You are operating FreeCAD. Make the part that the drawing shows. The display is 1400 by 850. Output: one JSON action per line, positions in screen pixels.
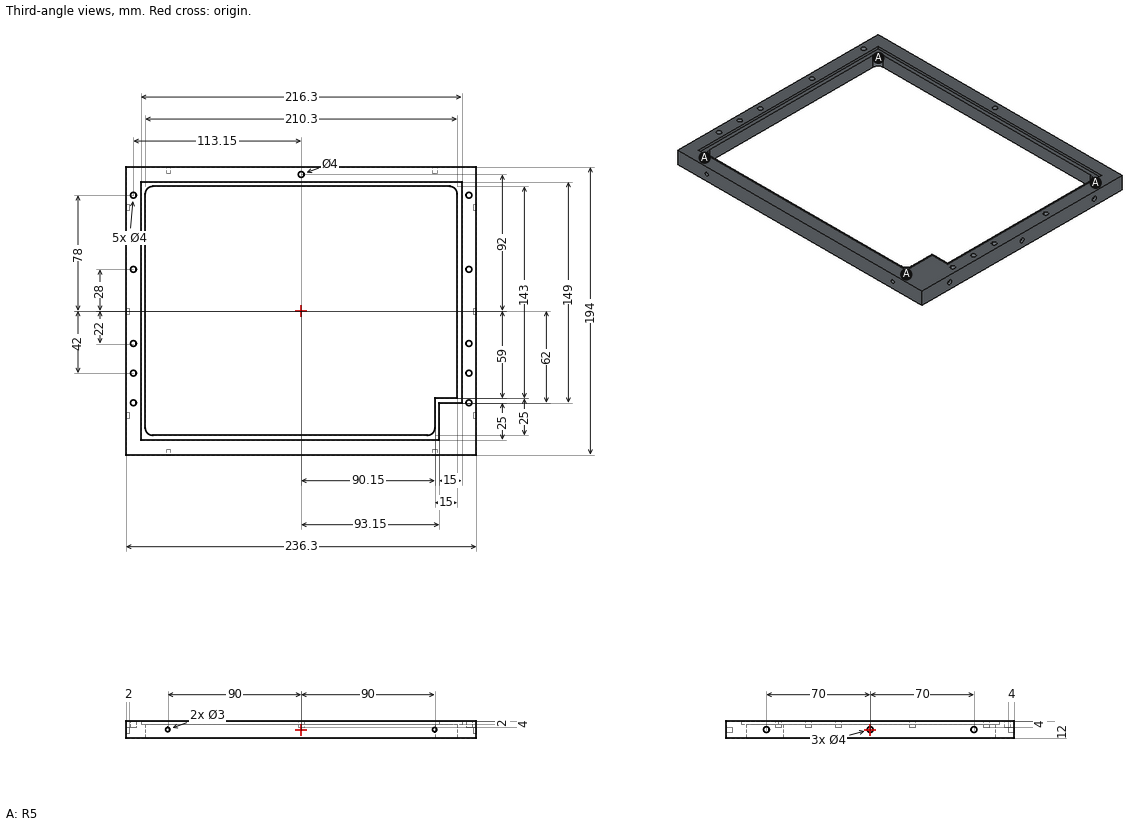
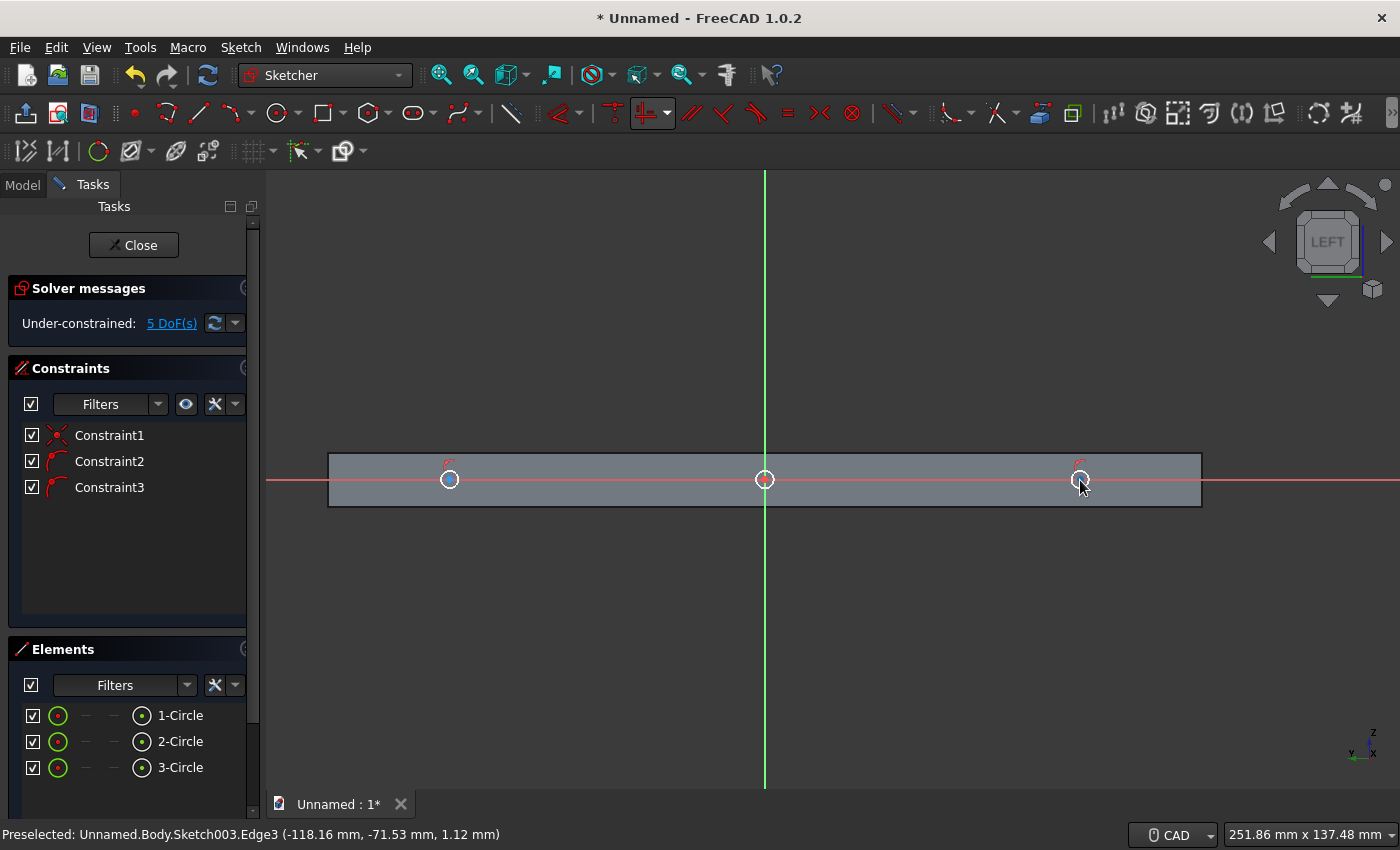
{"action": "scroll", "coordinate": [771, 473], "scroll_direction": "up", "scroll_amount": 5}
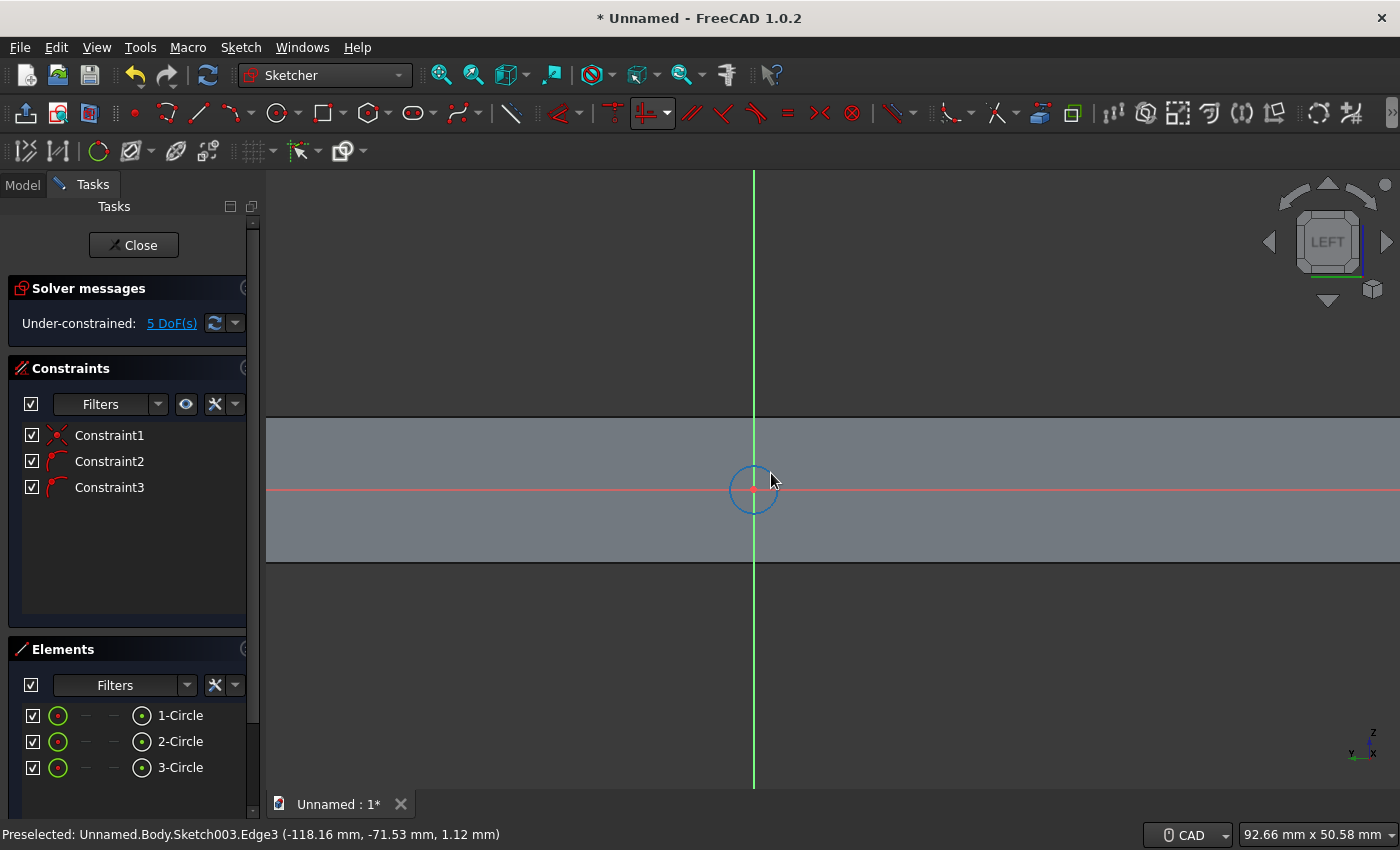
{"action": "left_click", "coordinate": [771, 473]}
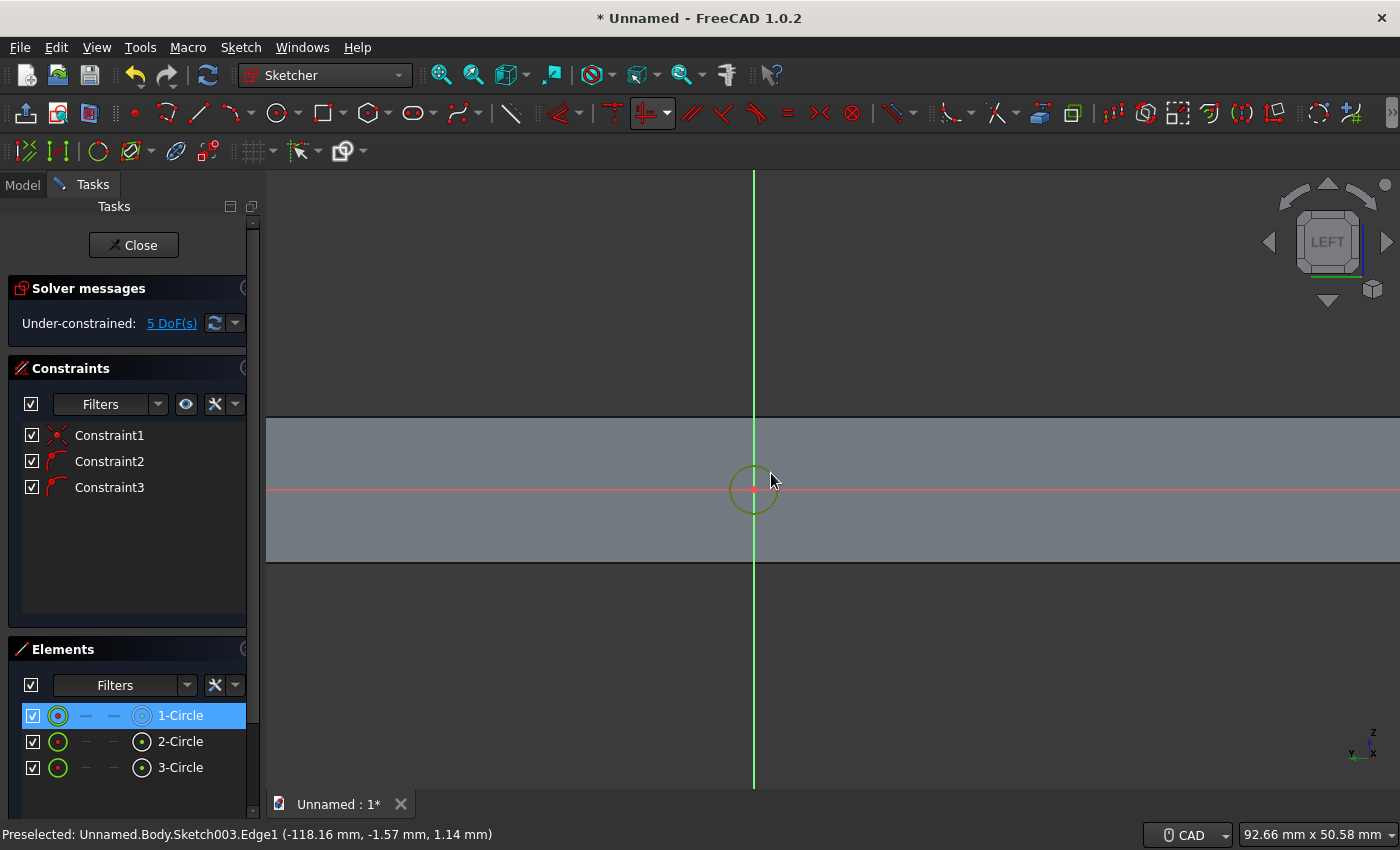
{"action": "scroll", "coordinate": [771, 473], "scroll_direction": "down", "scroll_amount": 5}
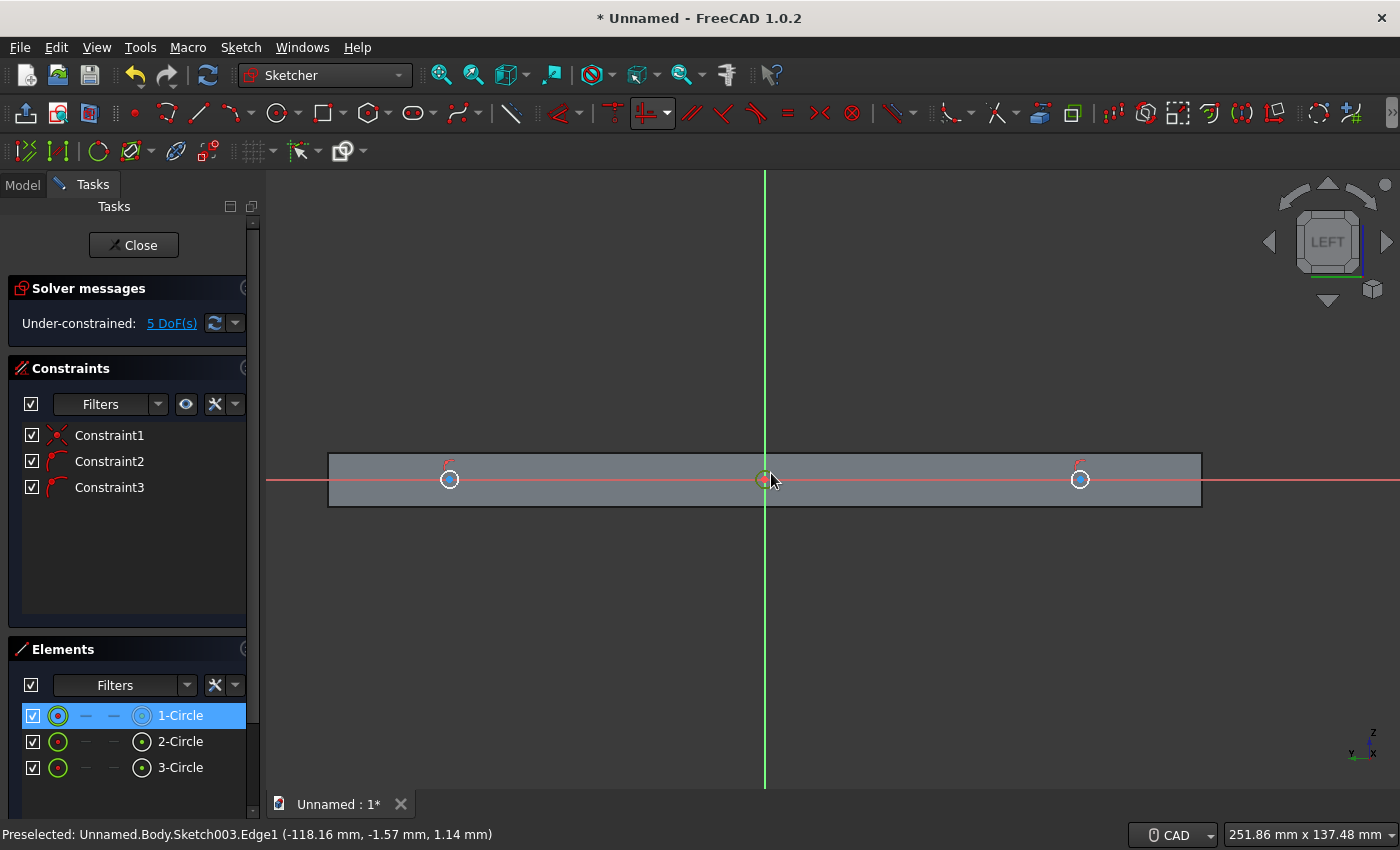
{"action": "scroll", "coordinate": [456, 473], "scroll_direction": "up", "scroll_amount": 5}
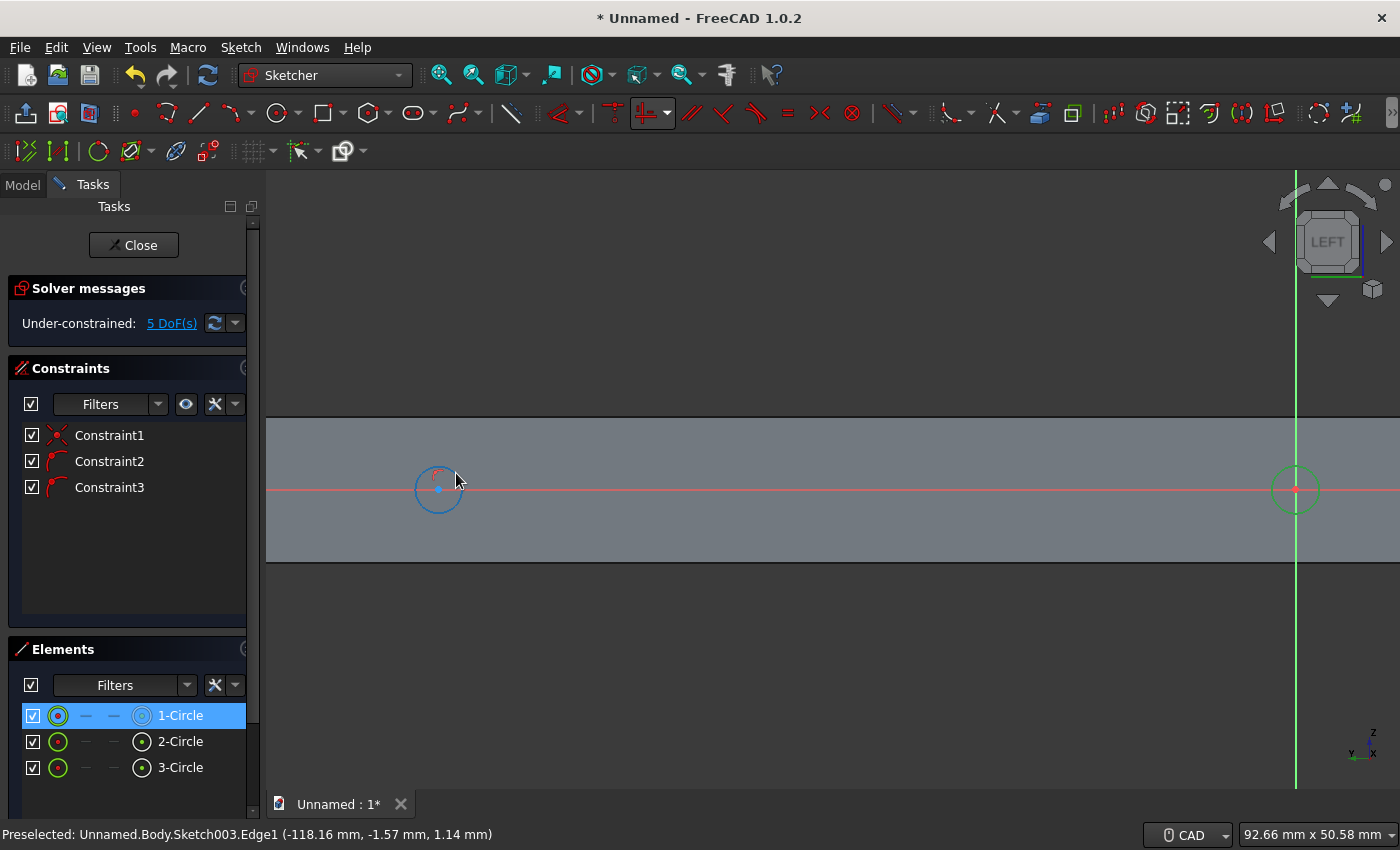
{"action": "left_click", "coordinate": [455, 473]}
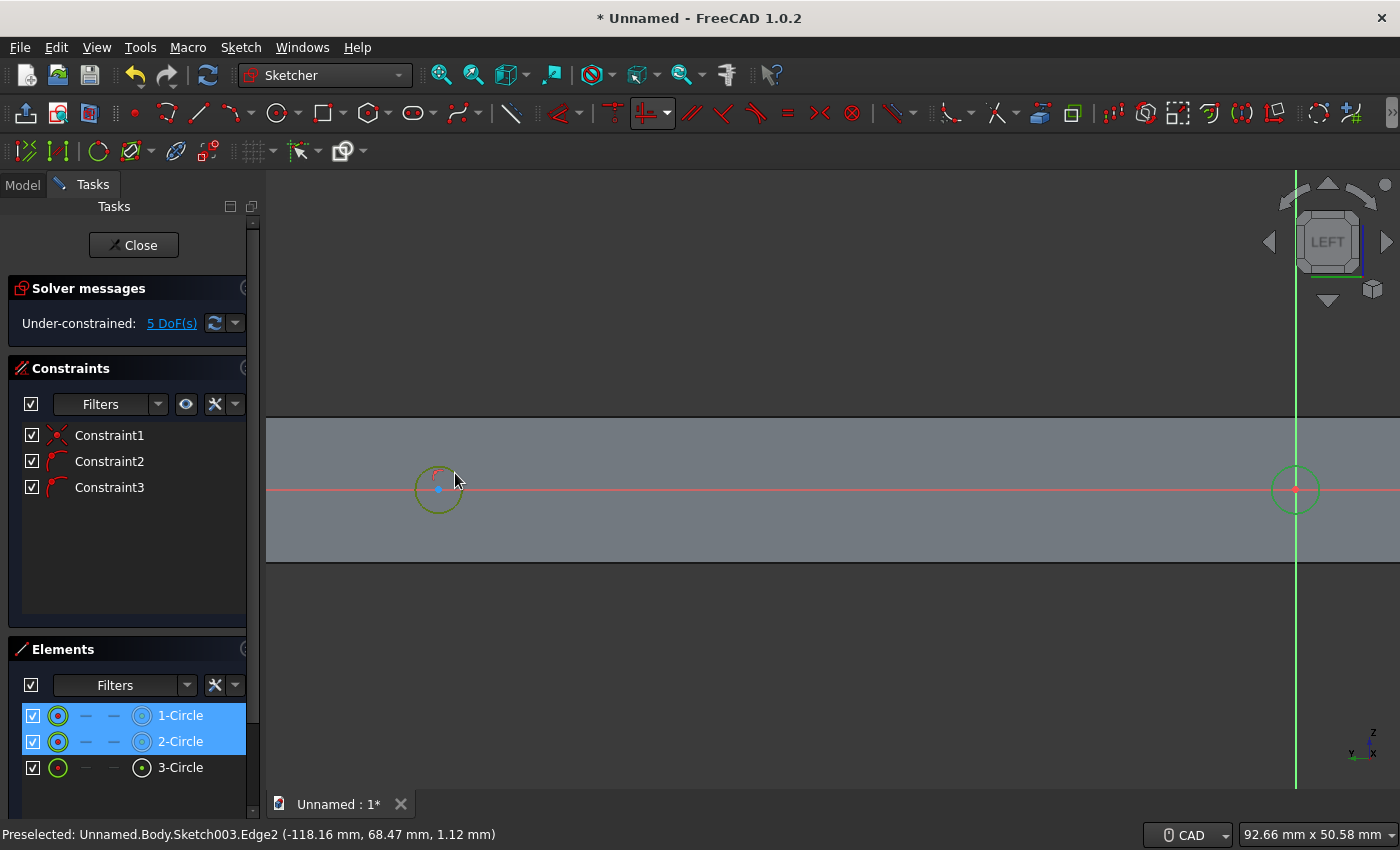
{"action": "scroll", "coordinate": [455, 473], "scroll_direction": "down", "scroll_amount": 5}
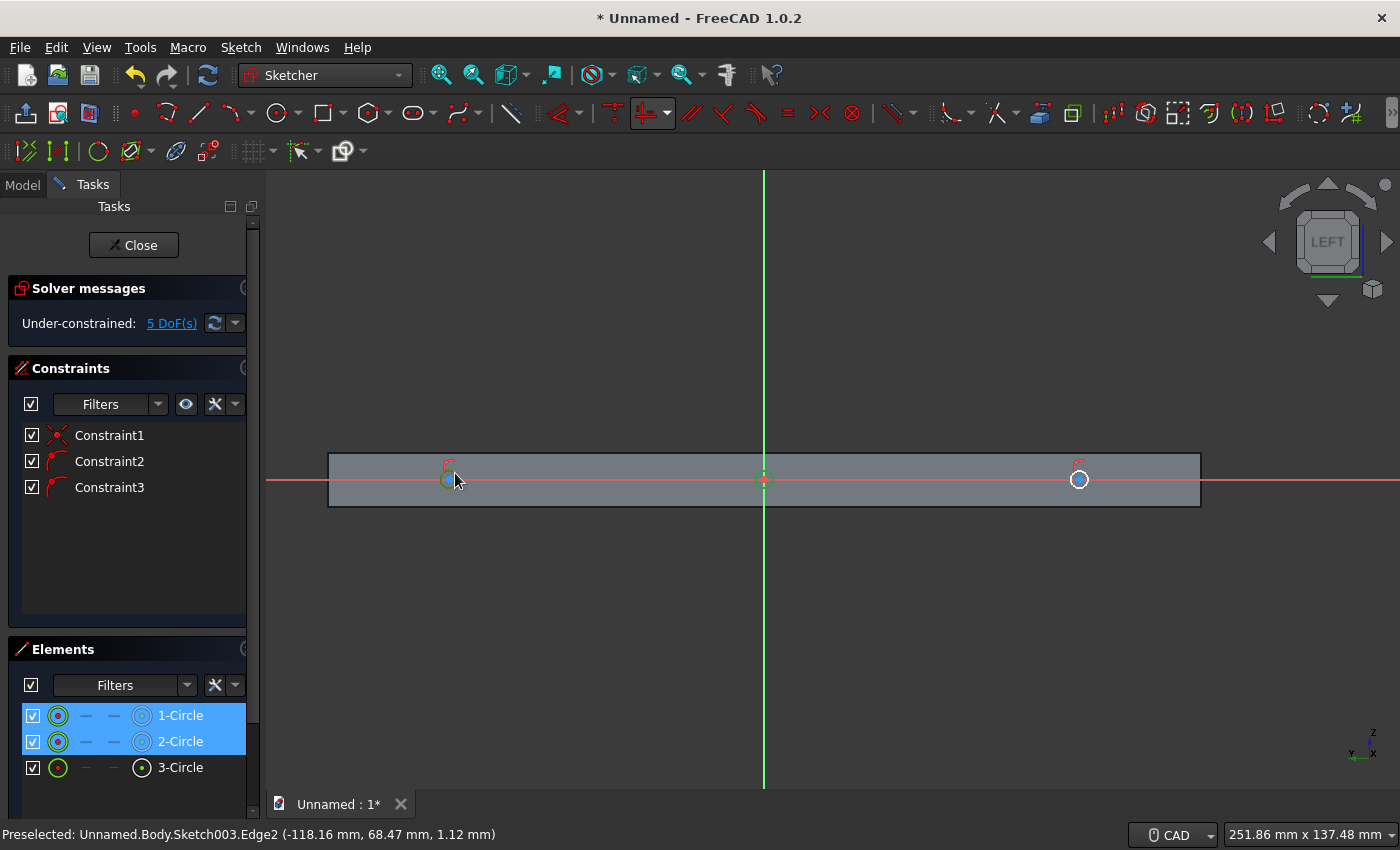
{"action": "scroll", "coordinate": [1085, 473], "scroll_direction": "up", "scroll_amount": 5}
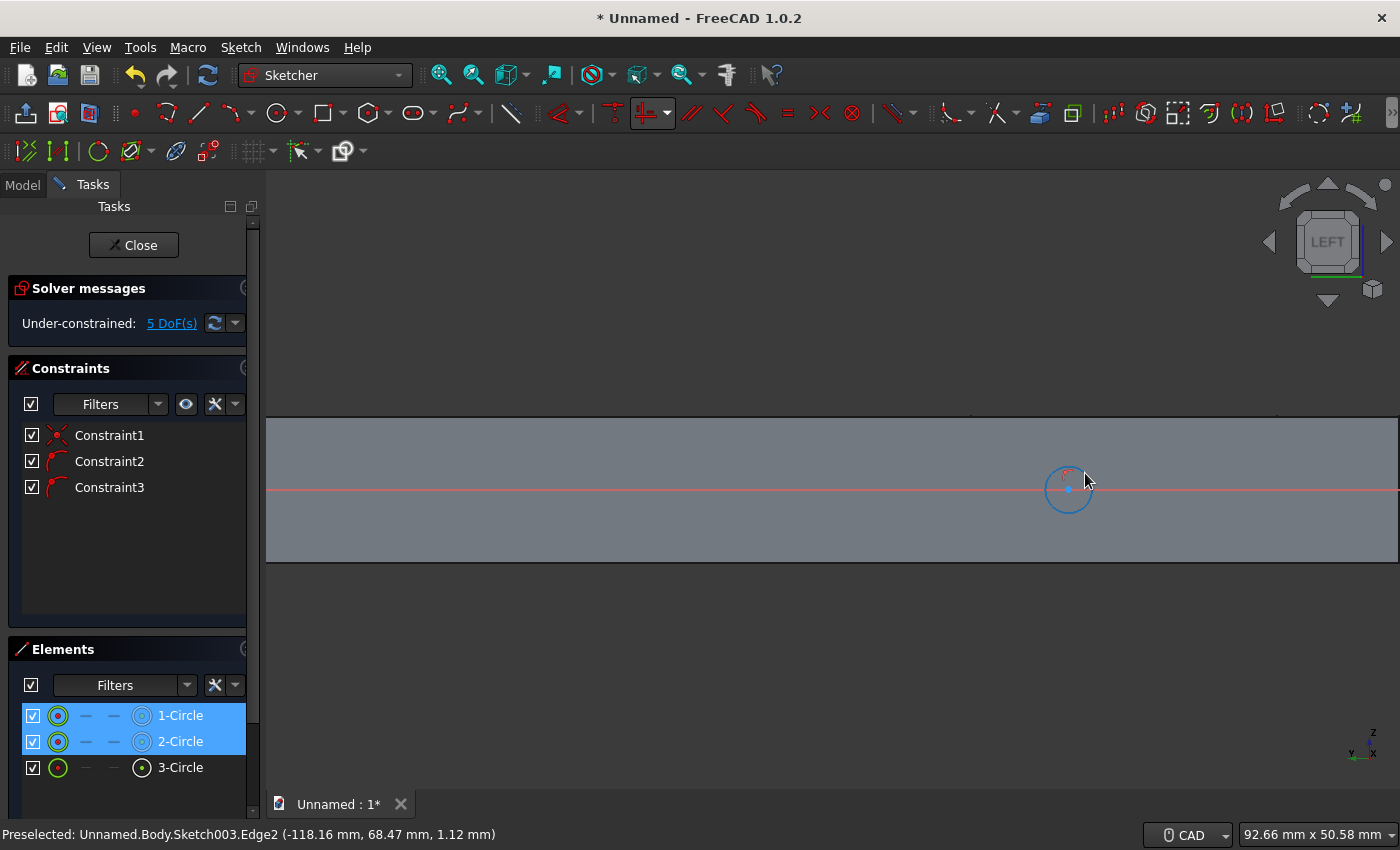
{"action": "left_click", "coordinate": [1085, 473]}